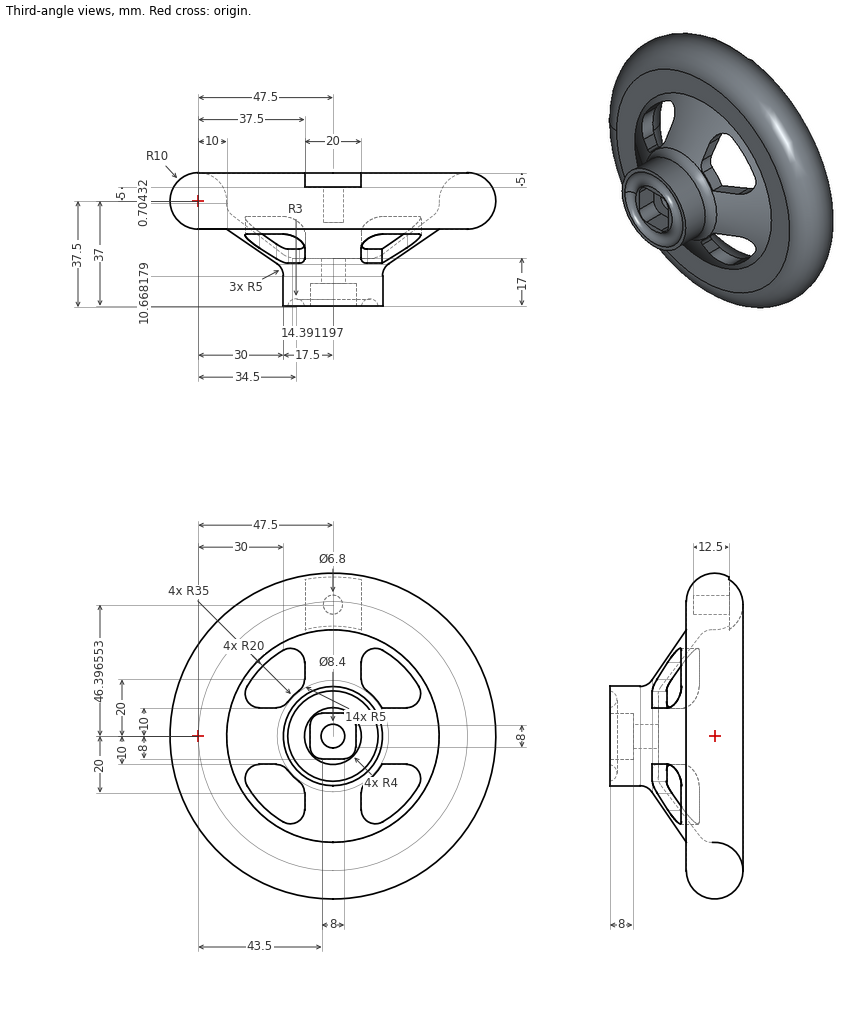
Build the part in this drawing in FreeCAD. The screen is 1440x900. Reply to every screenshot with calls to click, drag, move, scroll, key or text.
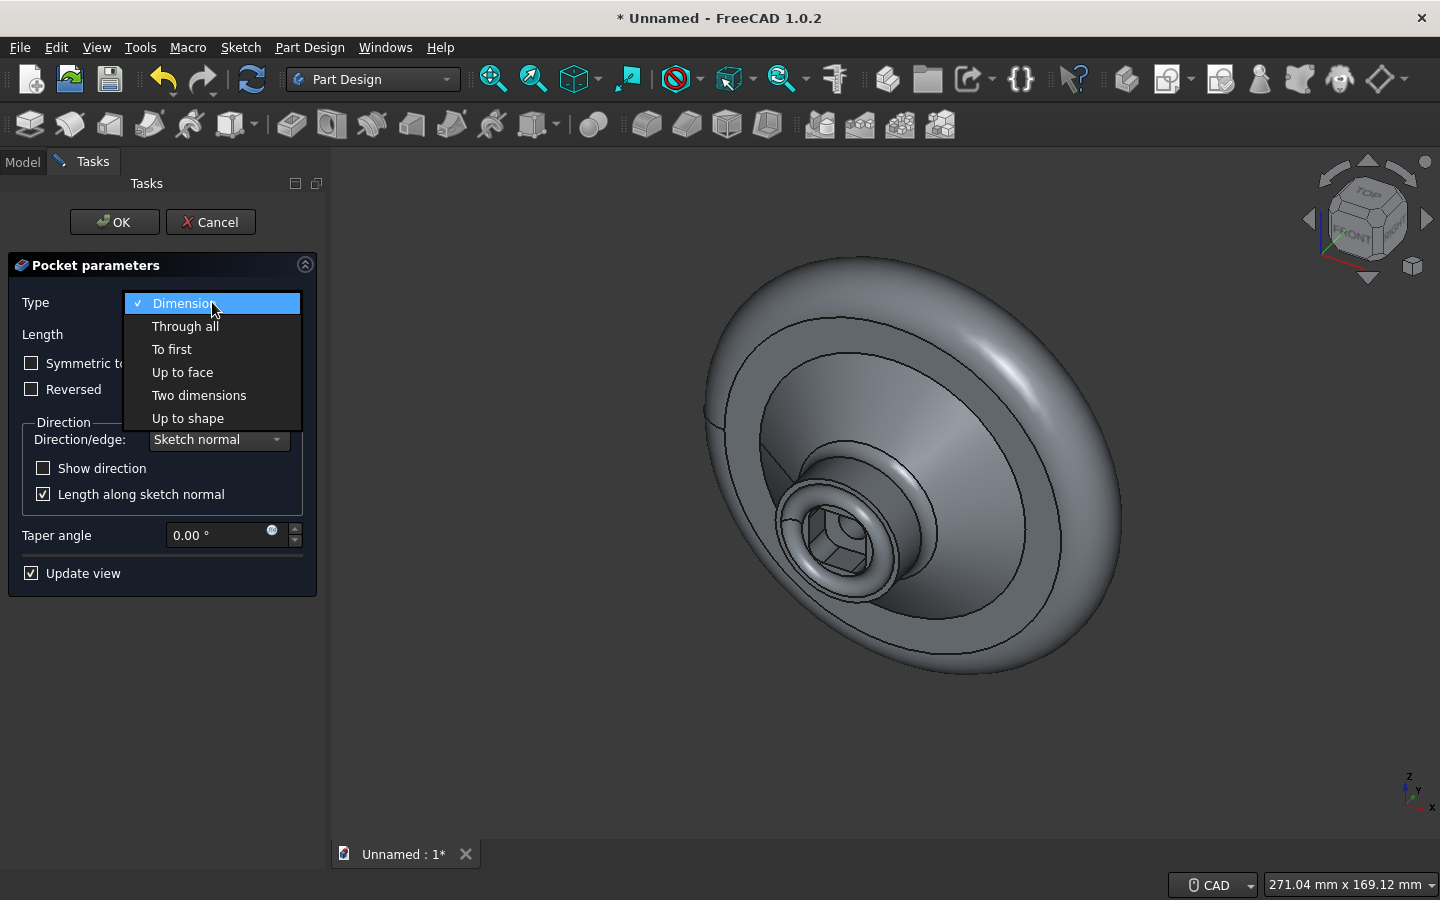
click(212, 326)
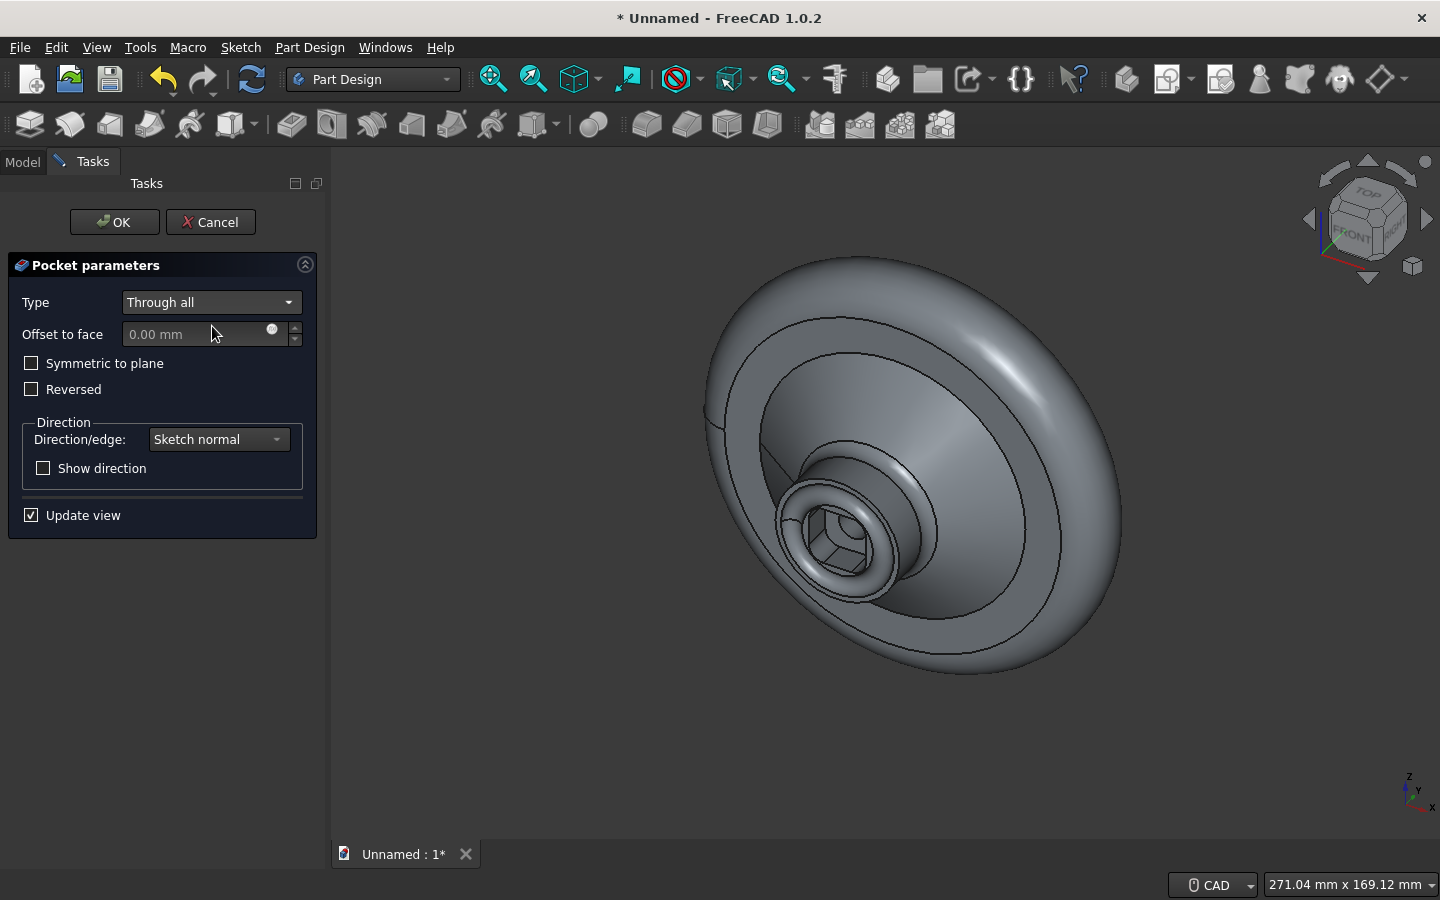
click(30, 389)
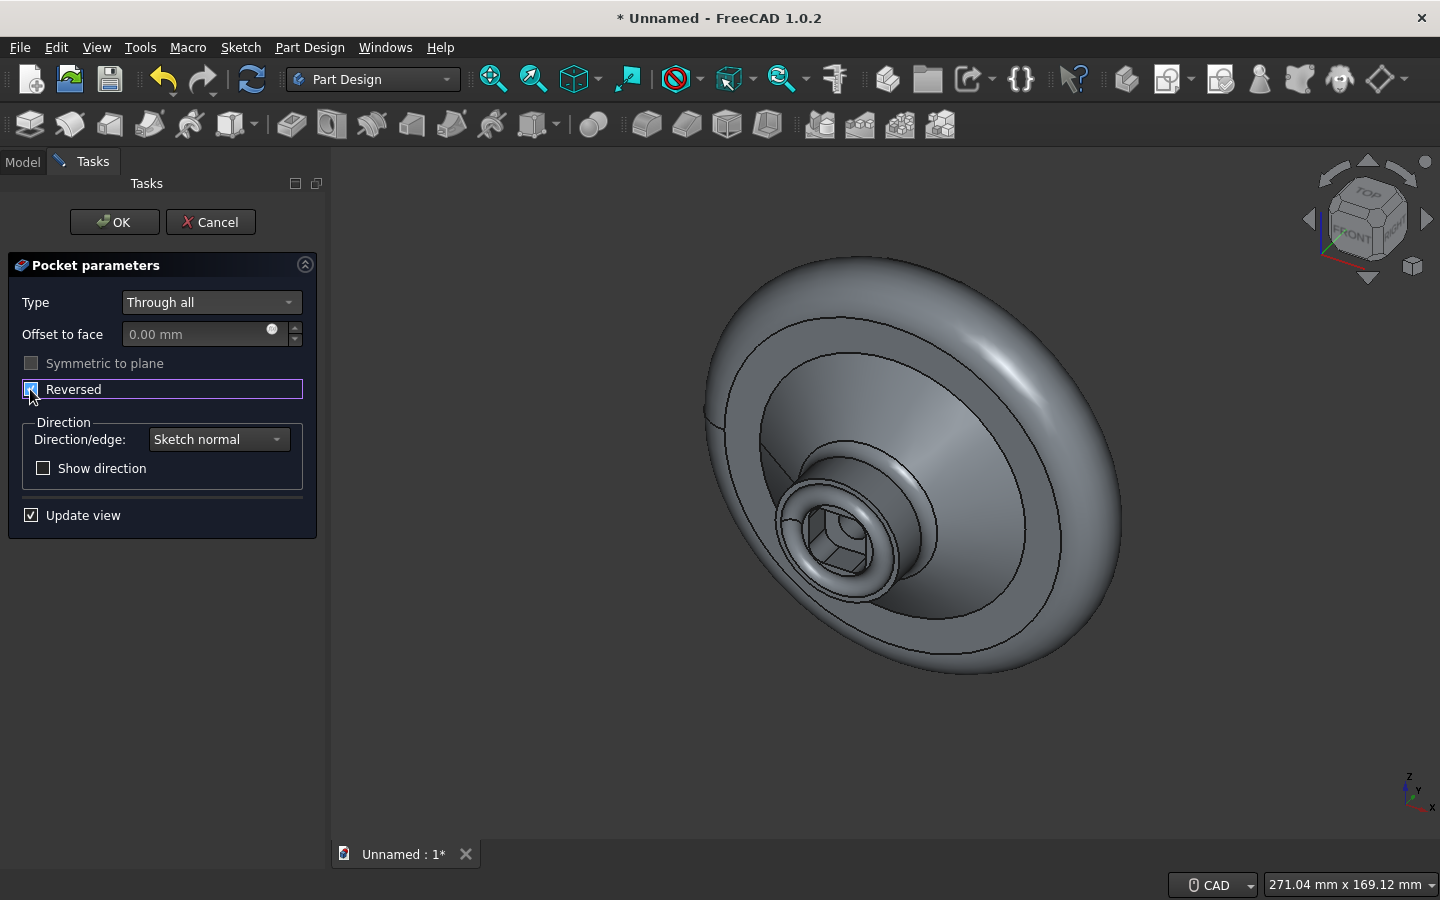
click(115, 222)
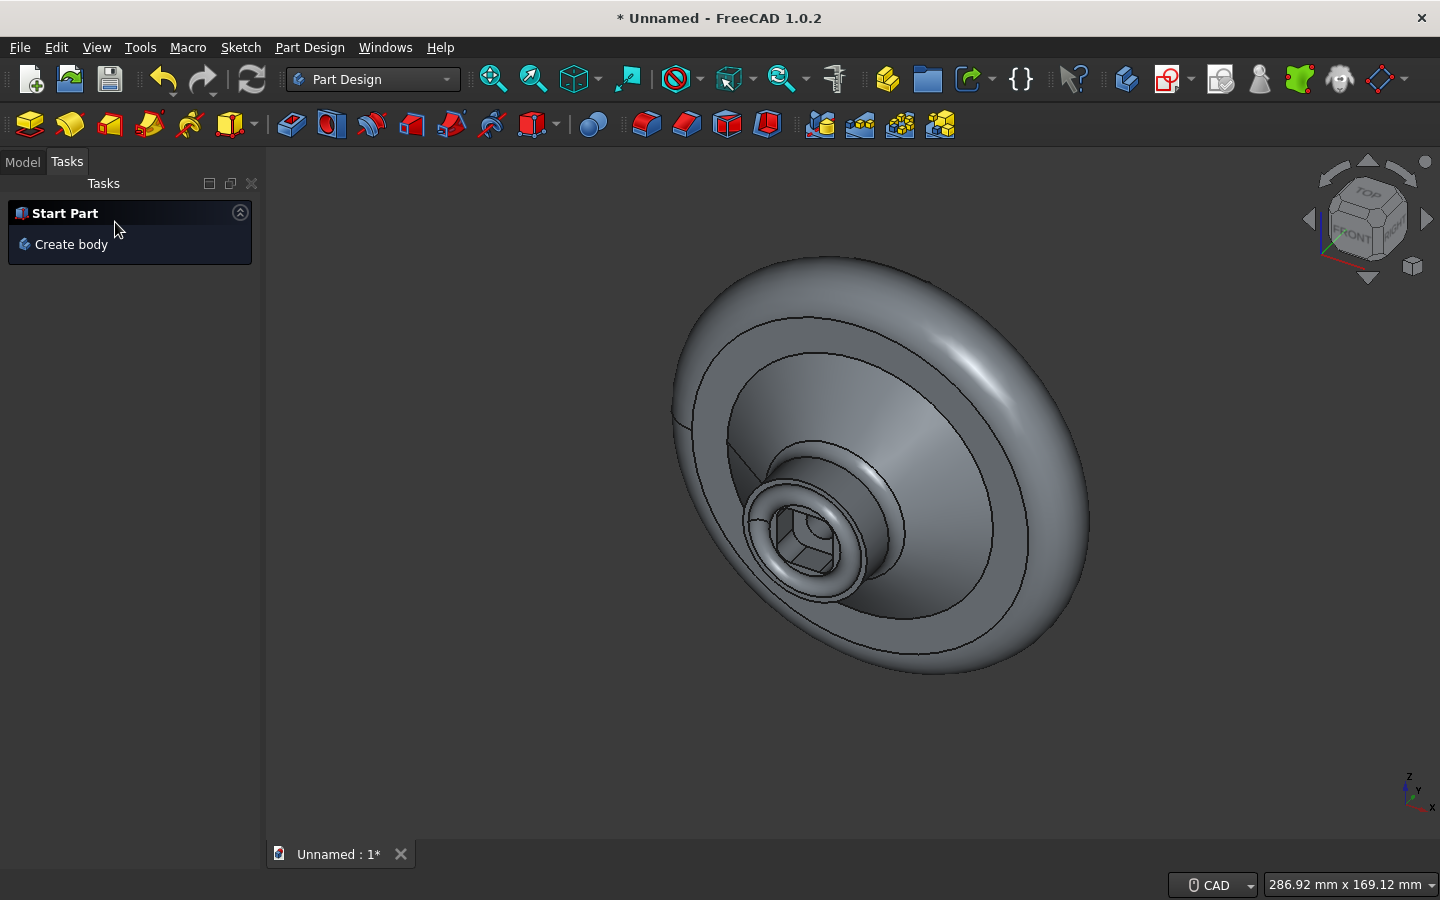
click(1168, 80)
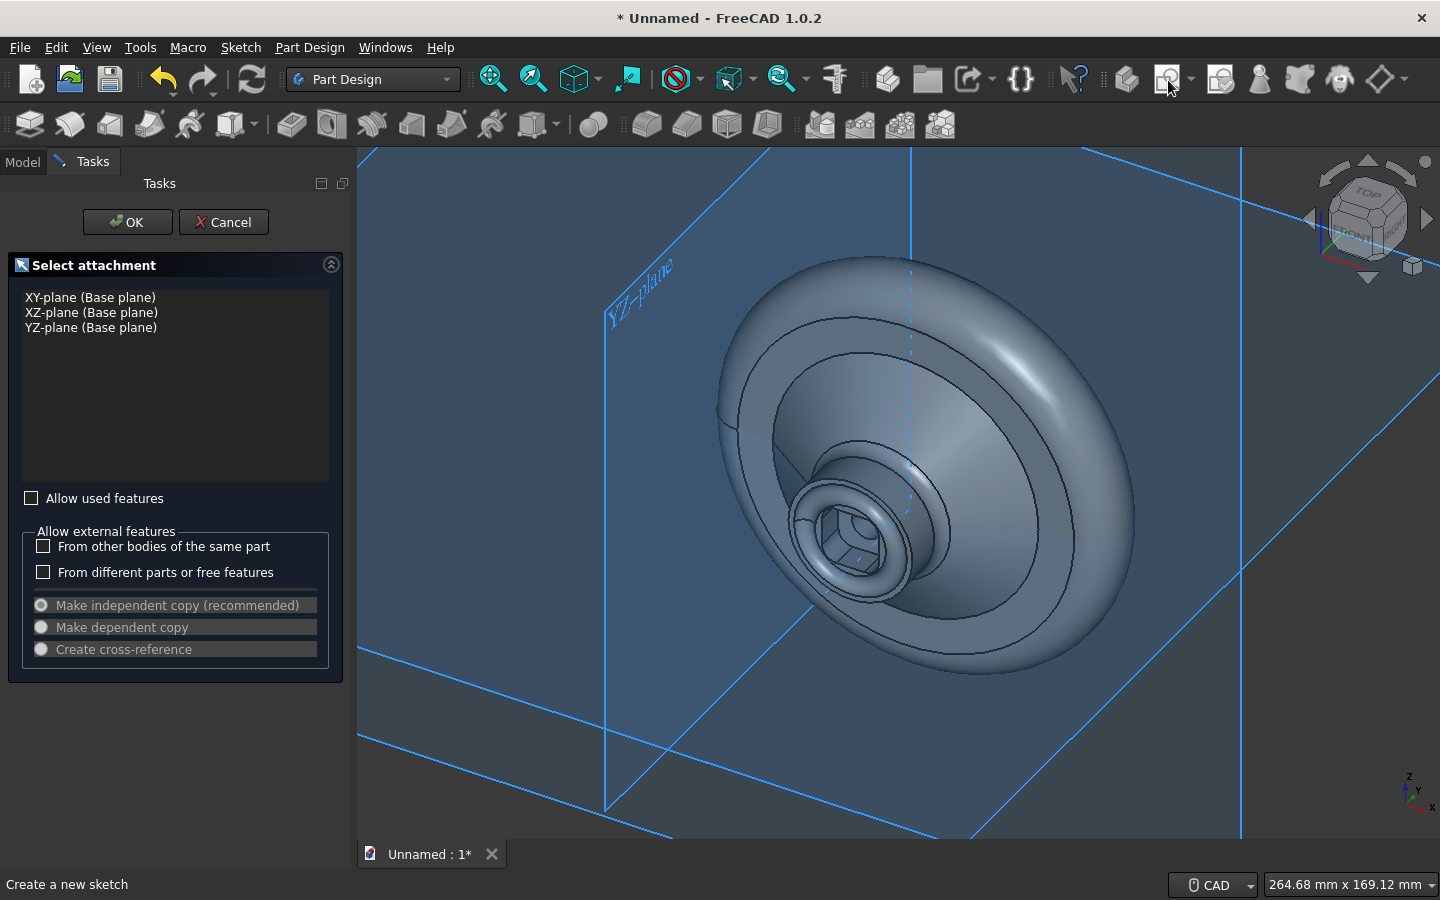
click(82, 312)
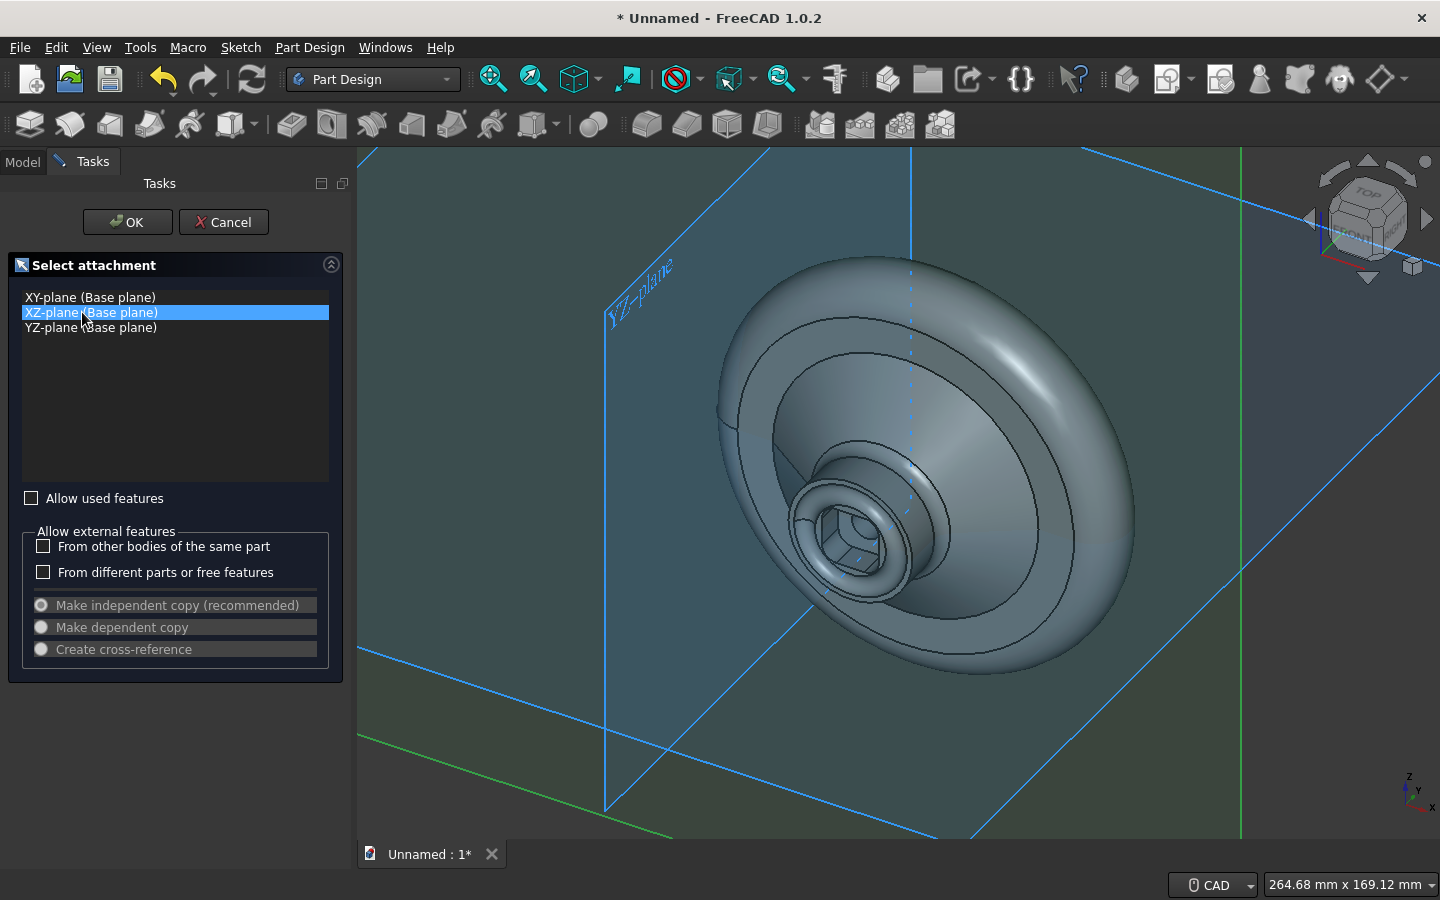
click(128, 222)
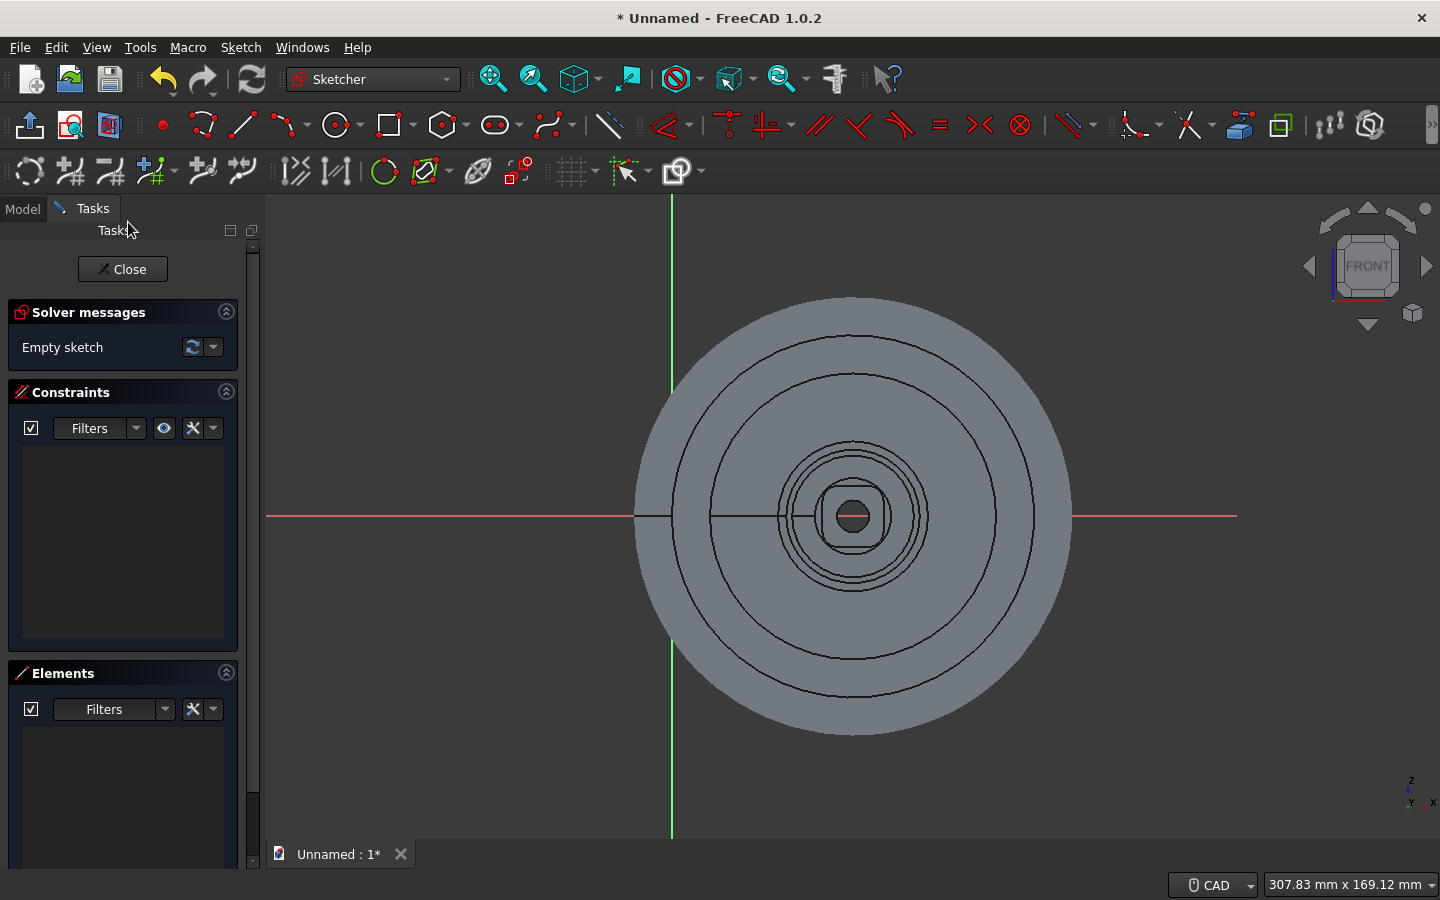
click(110, 126)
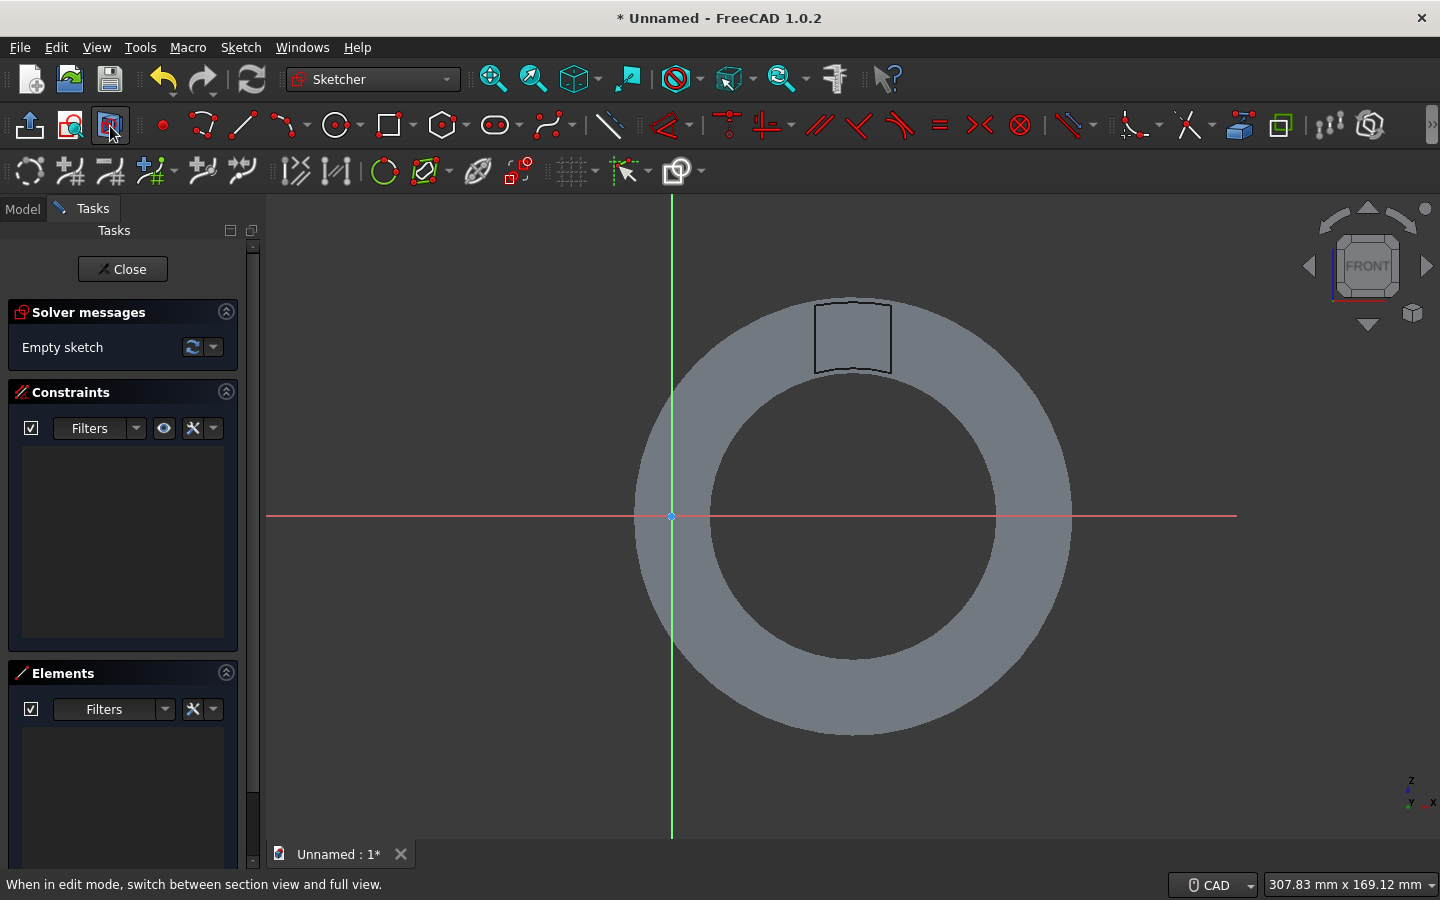
scroll(864, 516, up, 3)